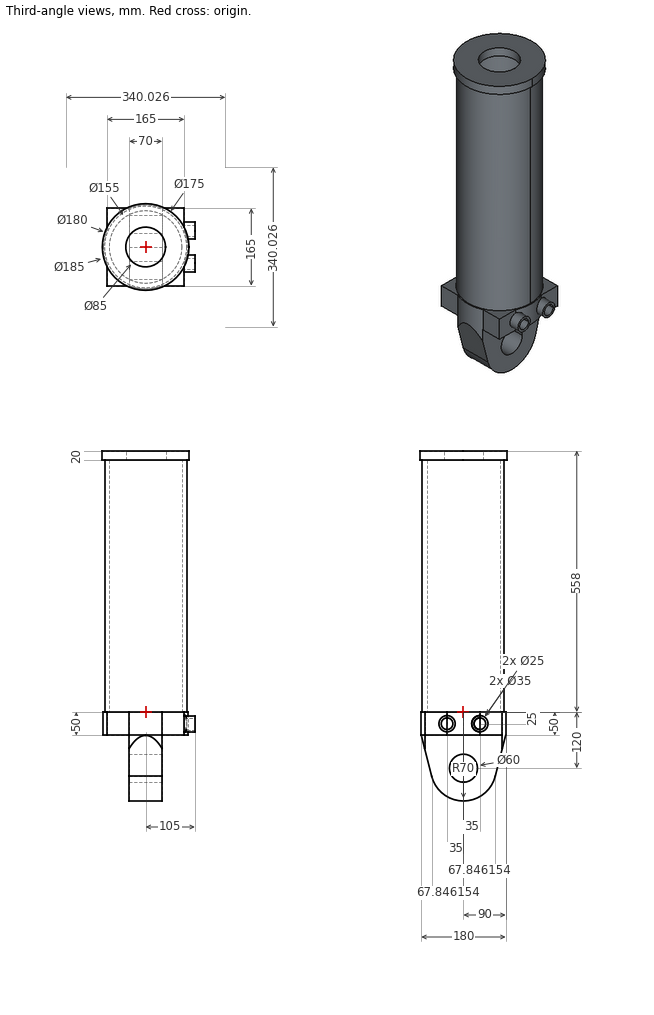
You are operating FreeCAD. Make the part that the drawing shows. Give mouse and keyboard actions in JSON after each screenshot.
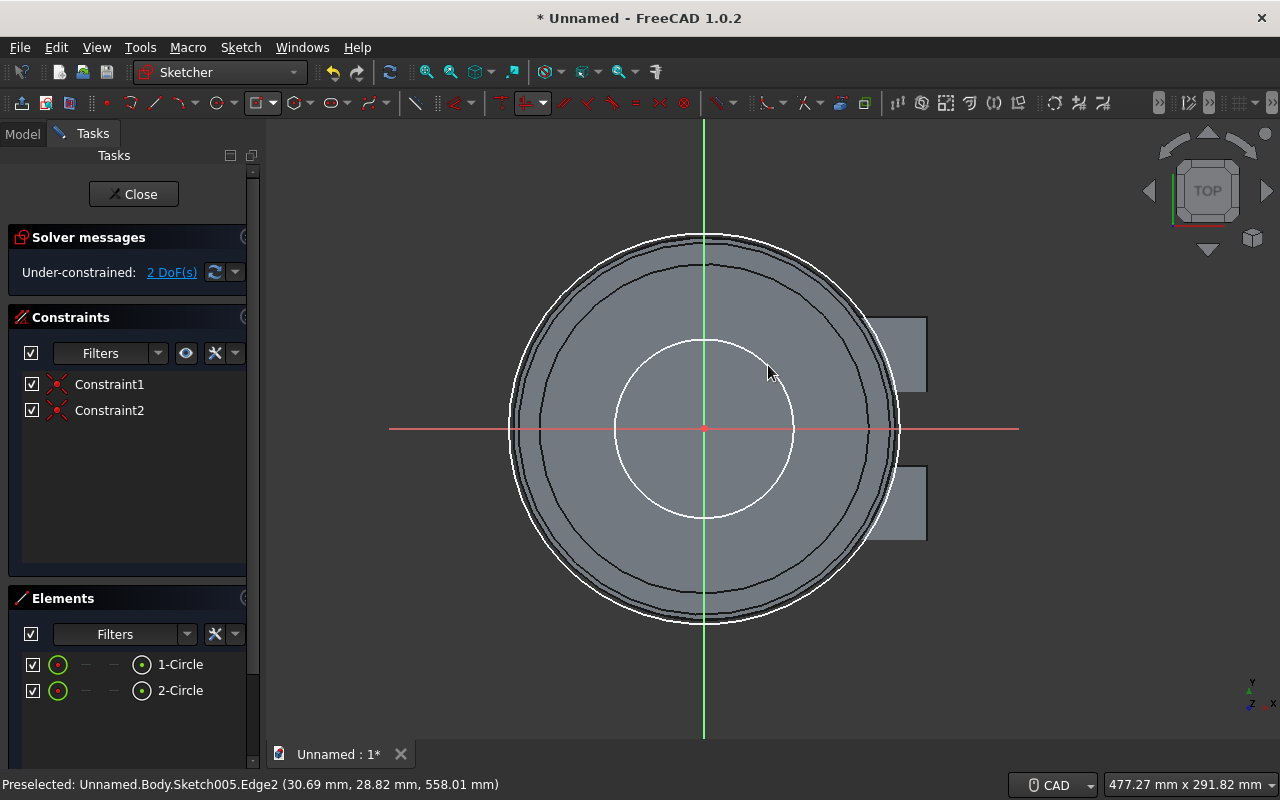
{"action": "left_click", "coordinate": [454, 104]}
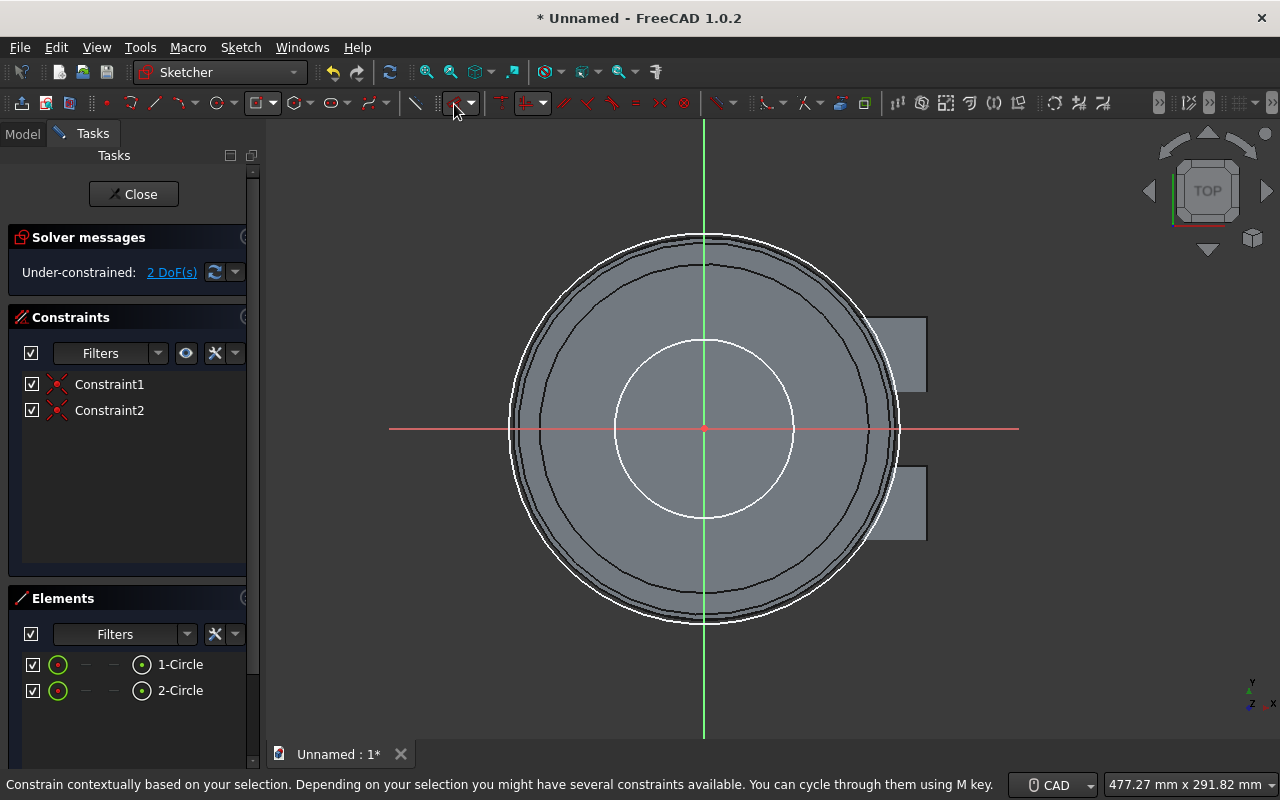
{"action": "left_click", "coordinate": [842, 290]}
{"action": "left_click", "coordinate": [865, 267]}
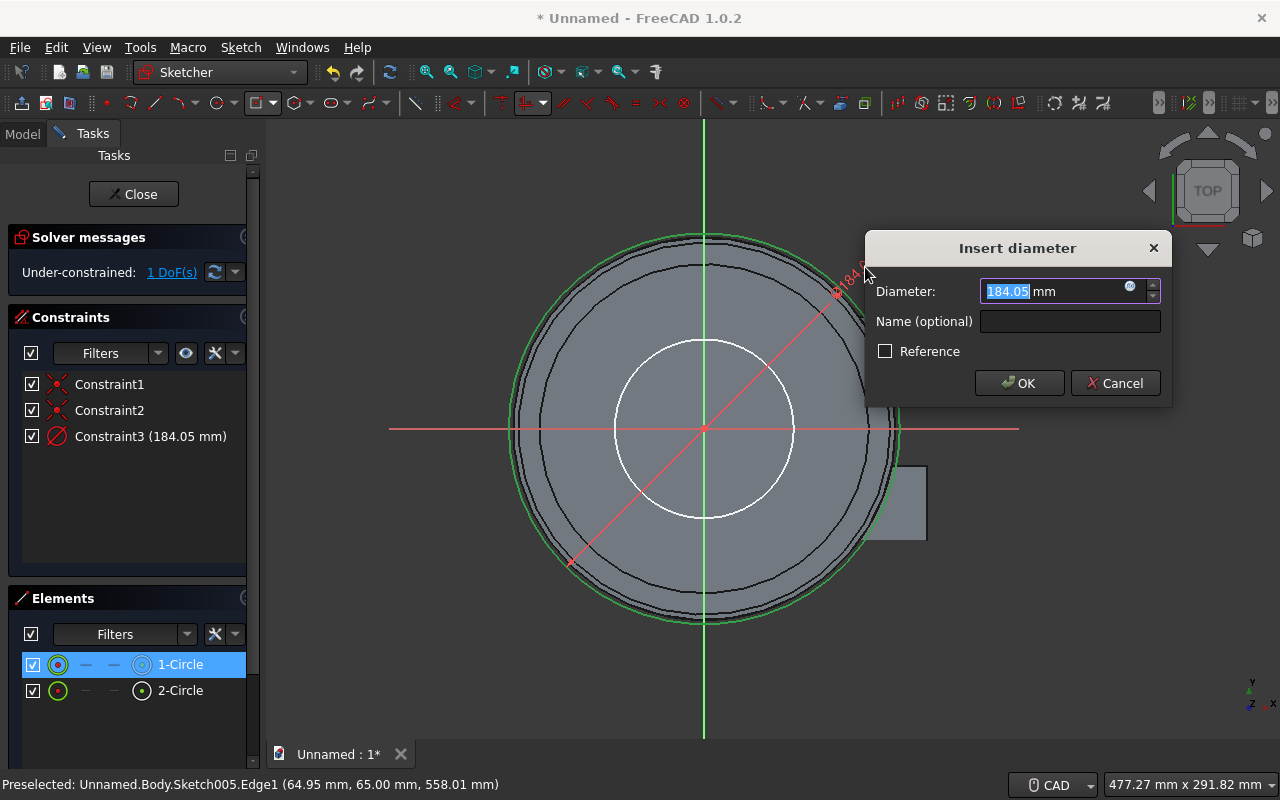
{"action": "type", "text": "185"}
{"action": "key", "text": "Return"}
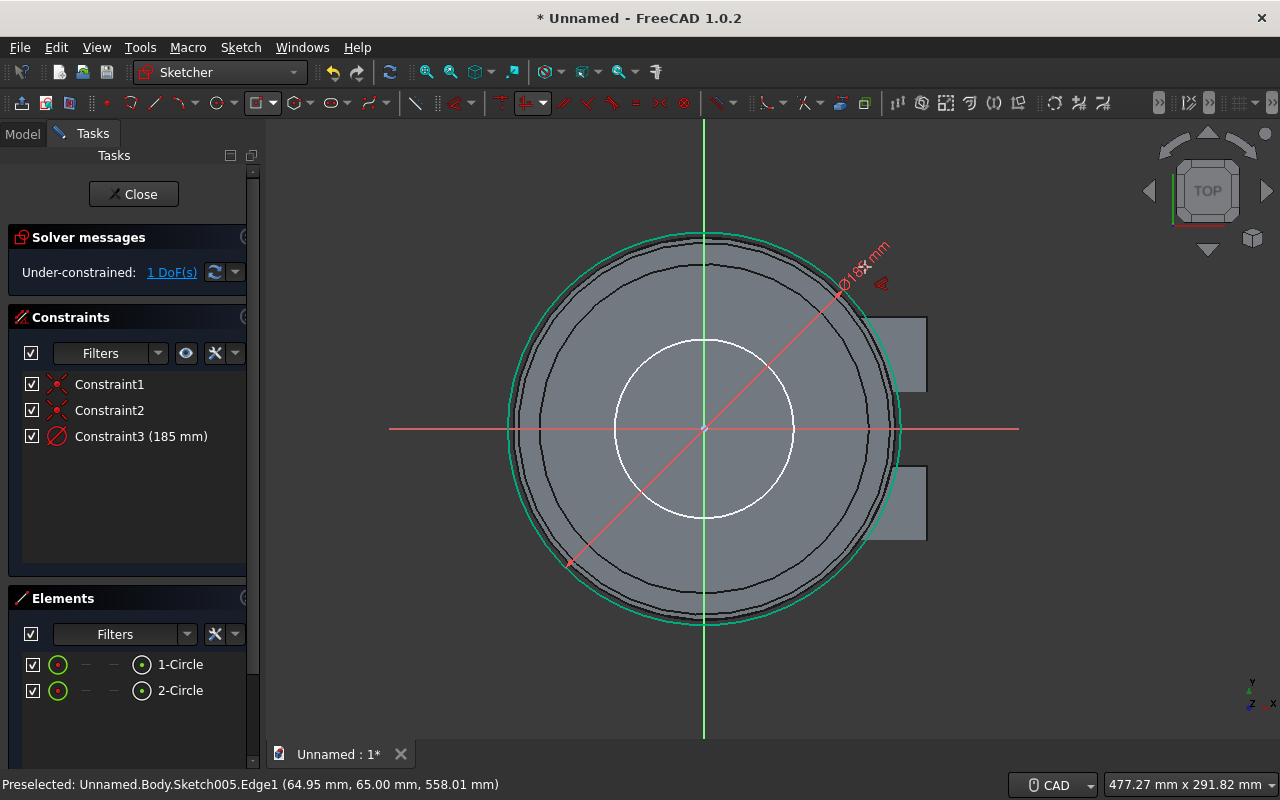
{"action": "left_click", "coordinate": [767, 365]}
{"action": "left_click", "coordinate": [789, 342]}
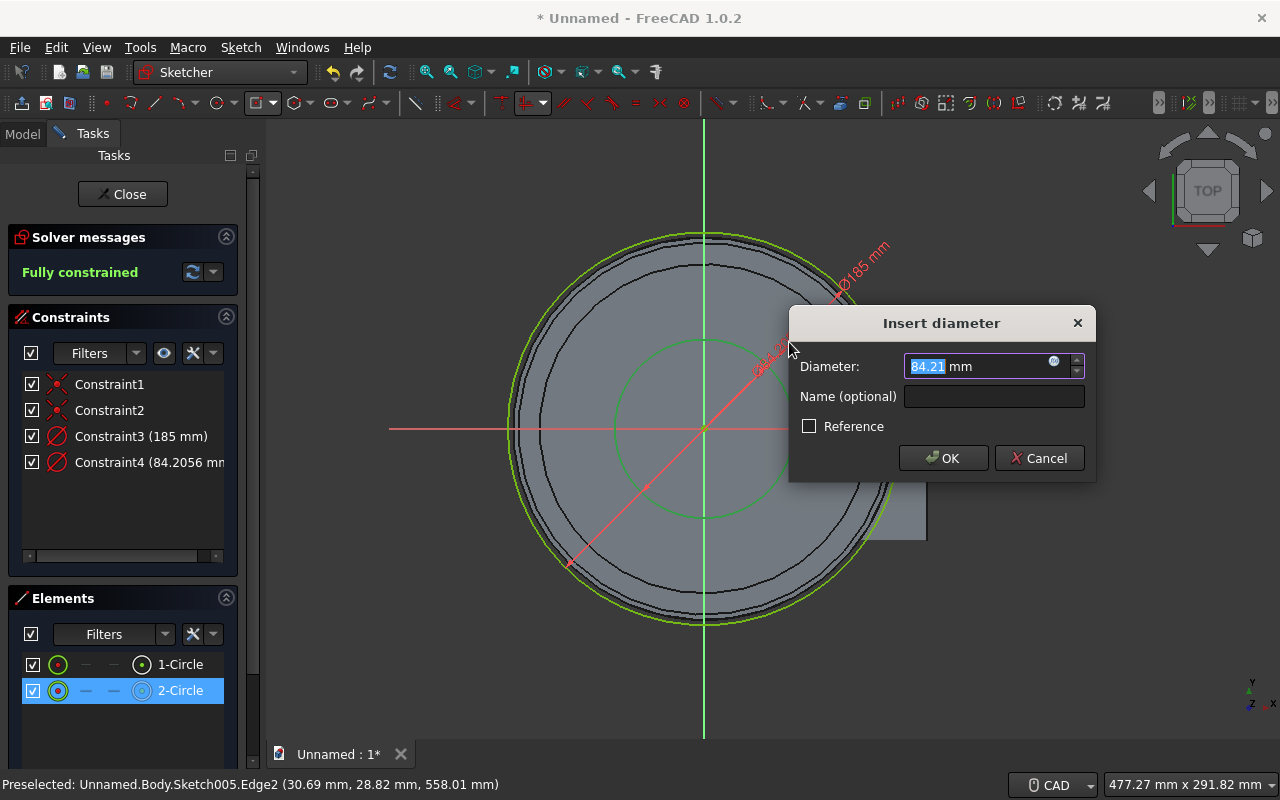
{"action": "type", "text": "85"}
{"action": "key", "text": "Return"}
{"action": "key", "text": "Escape"}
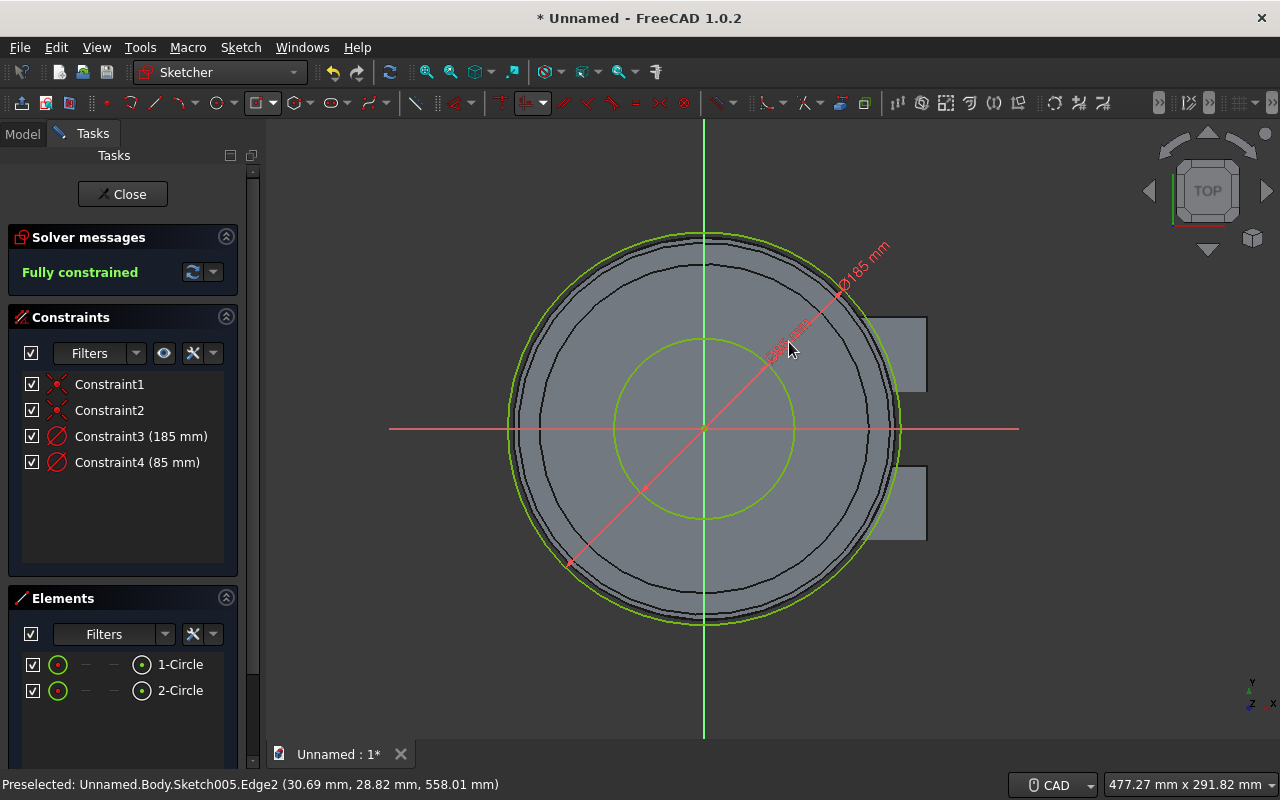
{"action": "left_click", "coordinate": [123, 194]}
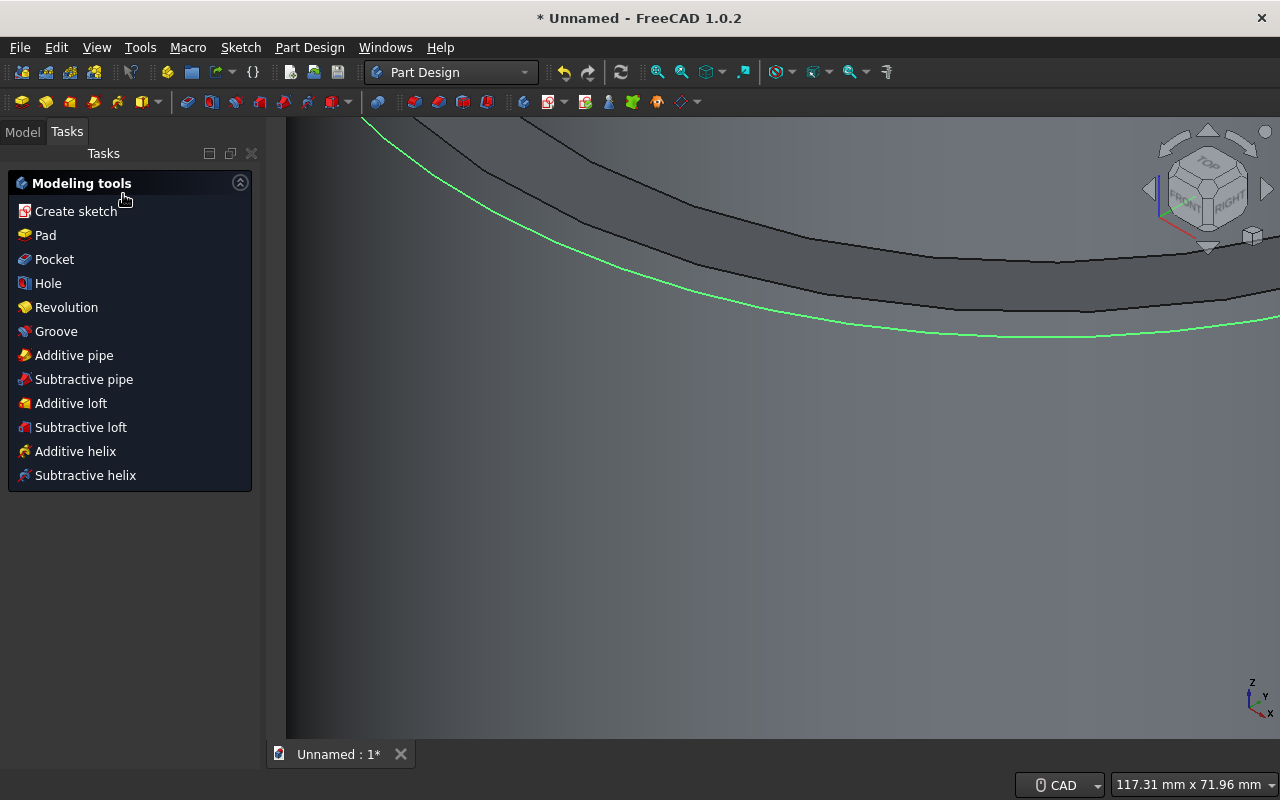
{"action": "left_click", "coordinate": [22, 102]}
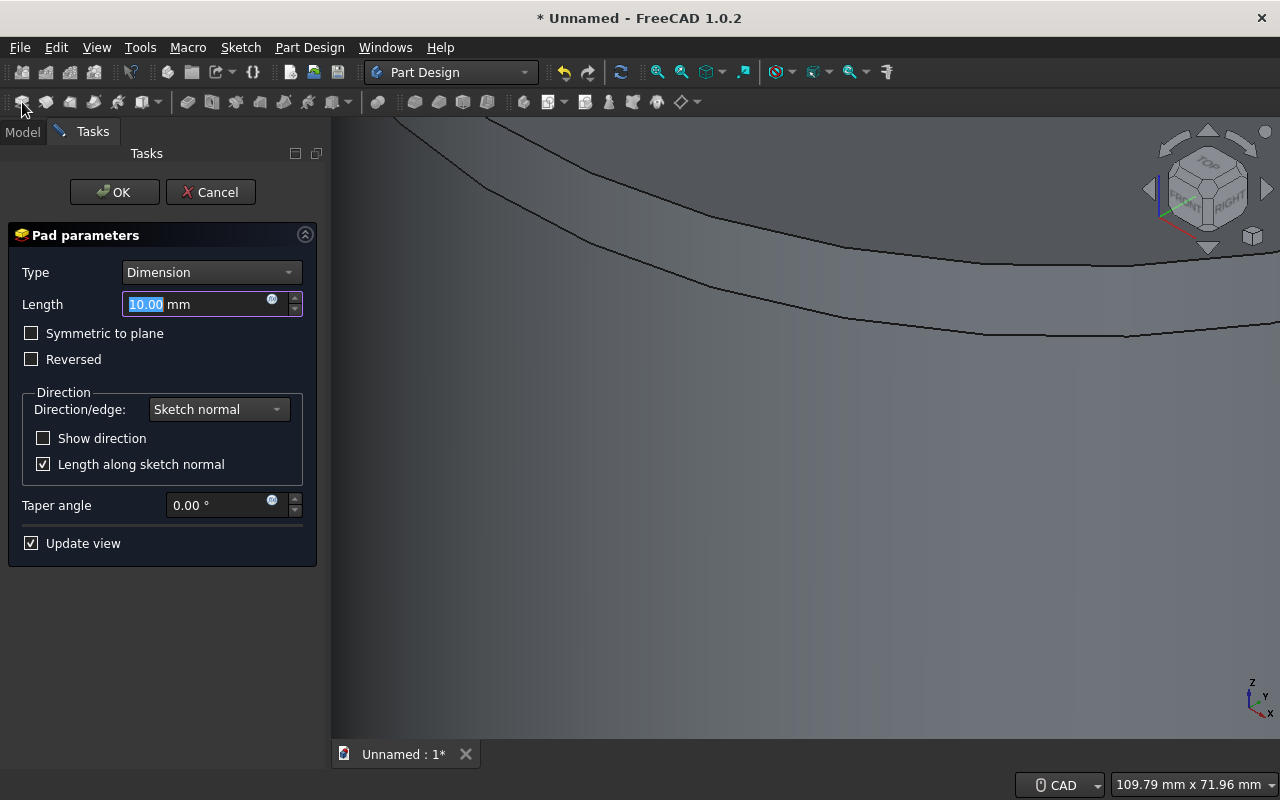
{"action": "type", "text": "20"}
{"action": "key", "text": "Tab"}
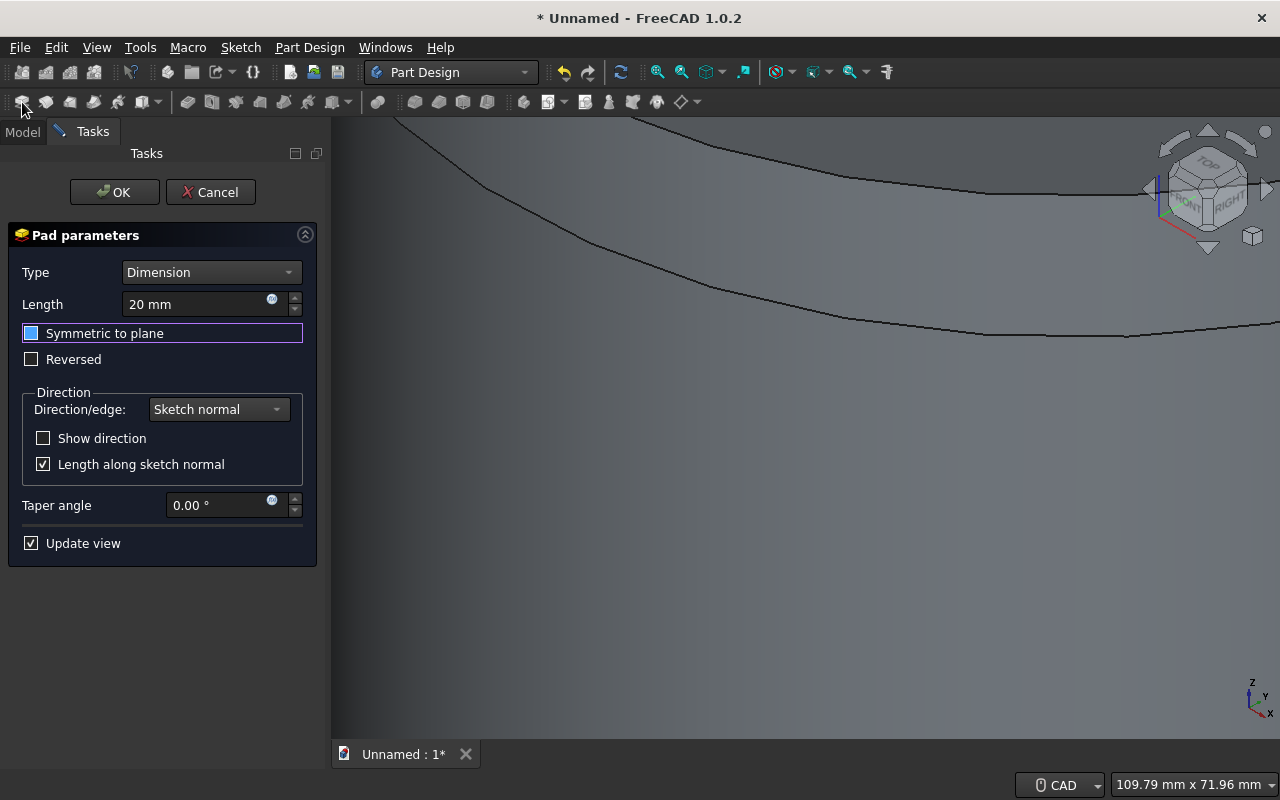
{"action": "left_click", "coordinate": [30, 359]}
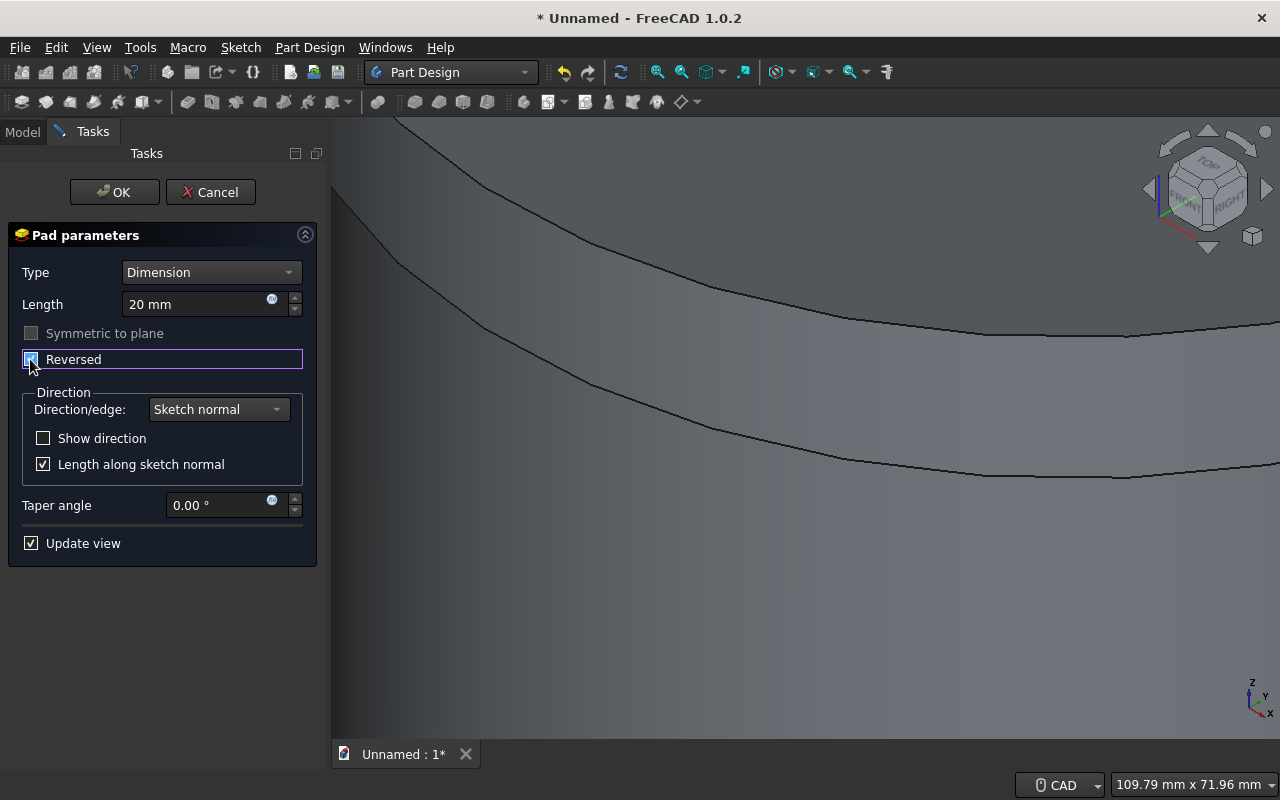
{"action": "left_click", "coordinate": [115, 192]}